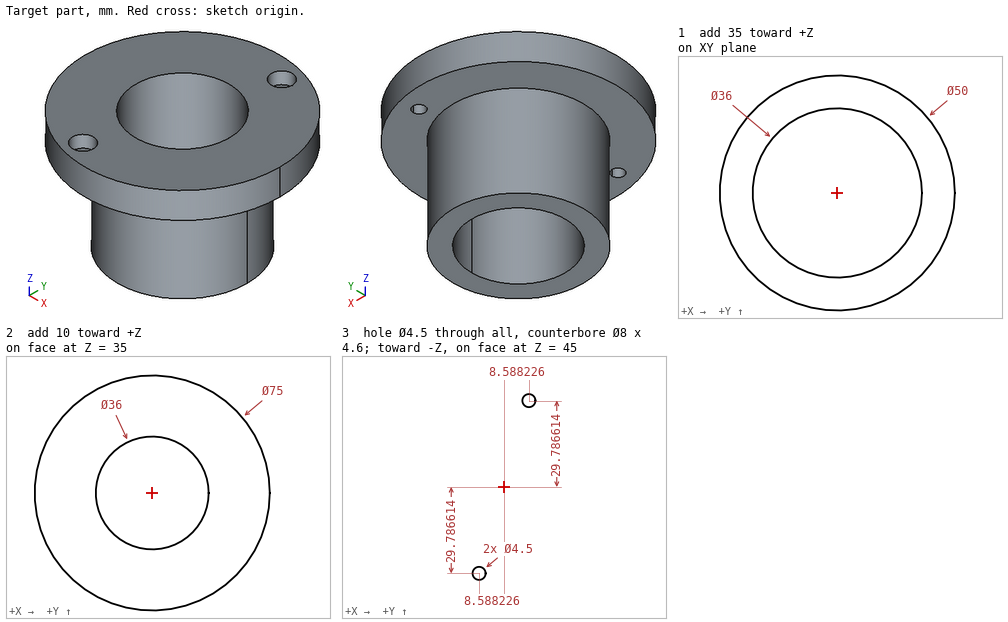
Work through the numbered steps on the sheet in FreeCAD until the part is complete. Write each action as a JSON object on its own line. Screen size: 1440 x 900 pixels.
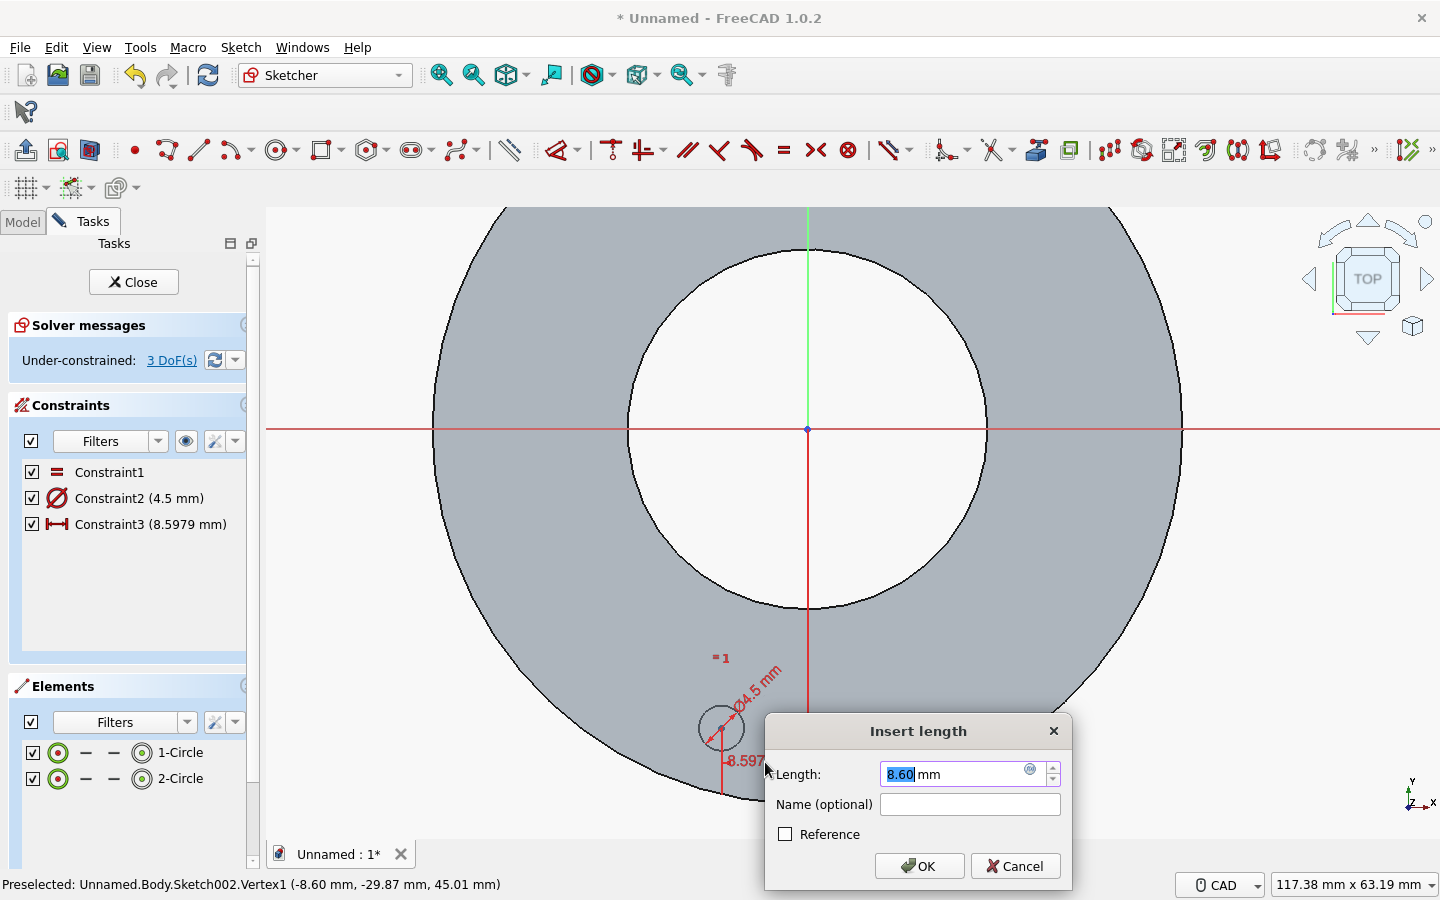
{"action": "type", "text": "8.588226"}
{"action": "key", "text": "Return"}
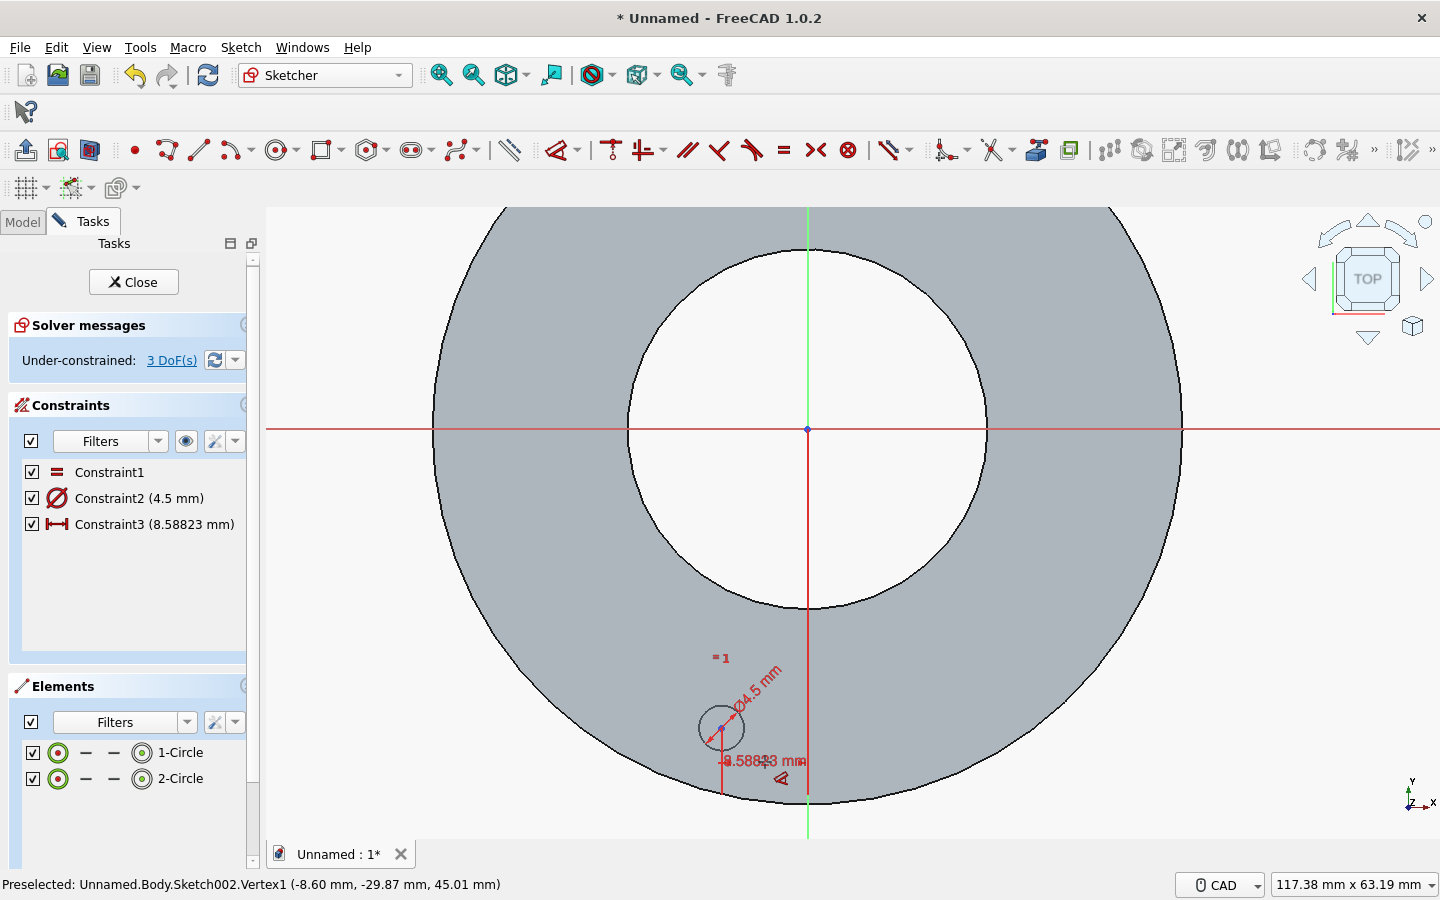
{"action": "scroll", "coordinate": [738, 713], "scroll_direction": "down", "scroll_amount": 2}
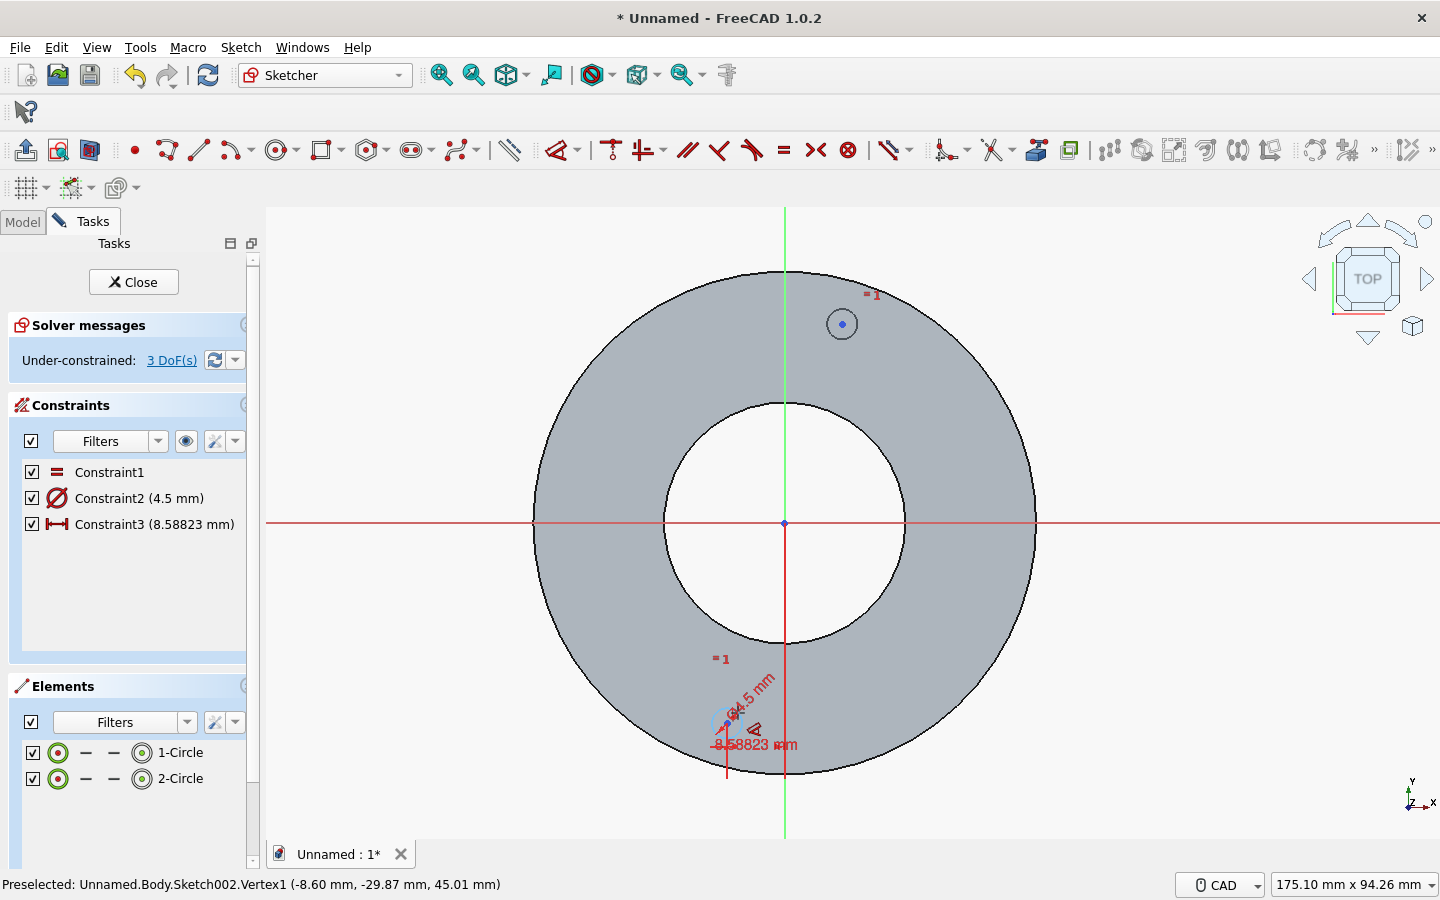
{"action": "left_click", "coordinate": [842, 324]}
{"action": "left_click", "coordinate": [813, 290]}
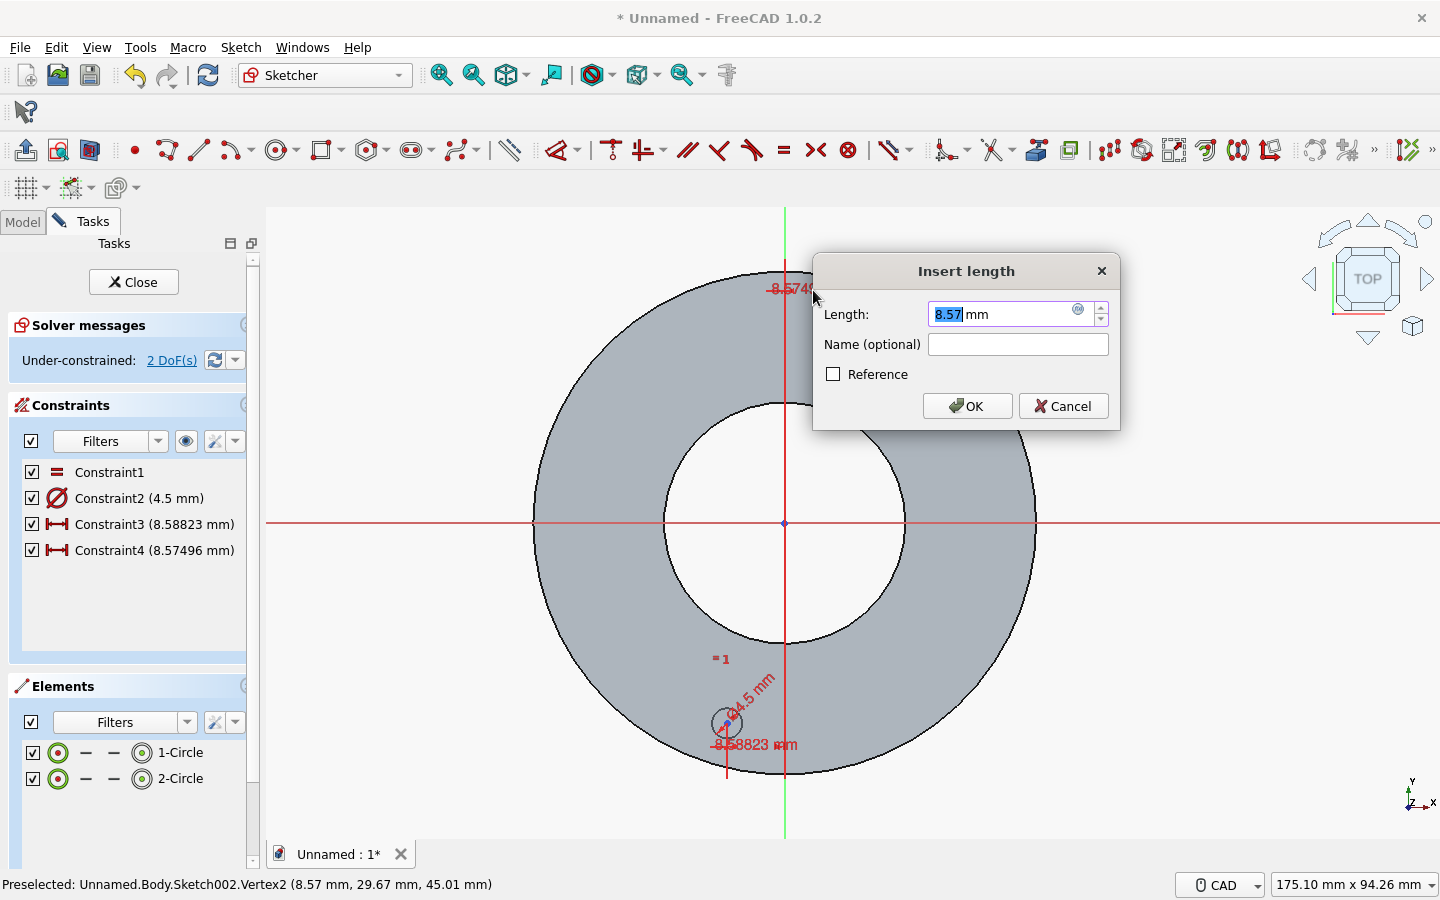
{"action": "type", "text": "8.588226"}
{"action": "key", "text": "Return"}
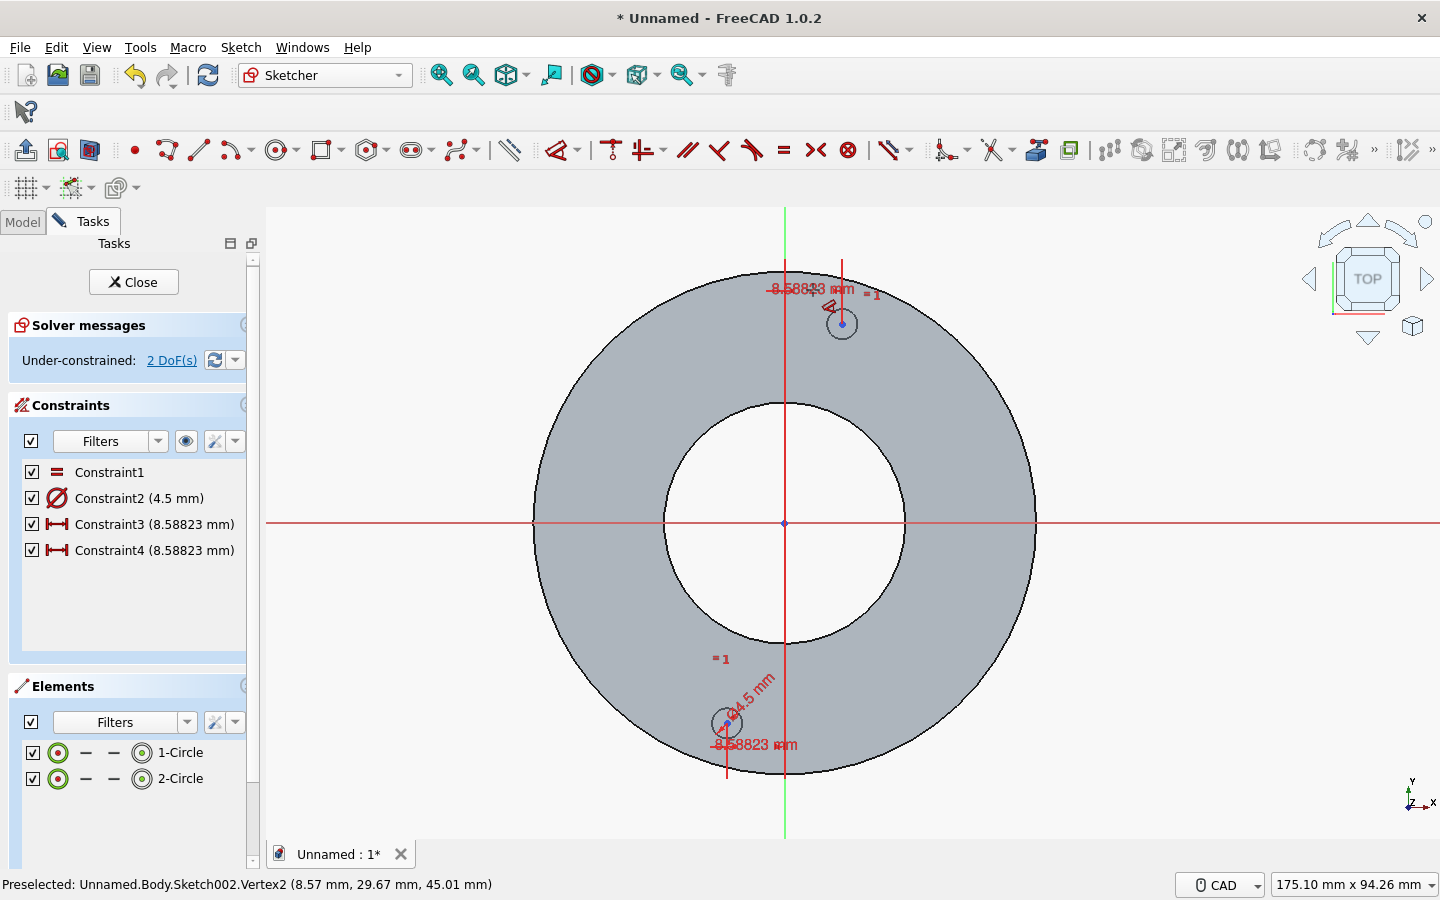
{"action": "left_click", "coordinate": [727, 723]}
{"action": "left_click", "coordinate": [693, 623]}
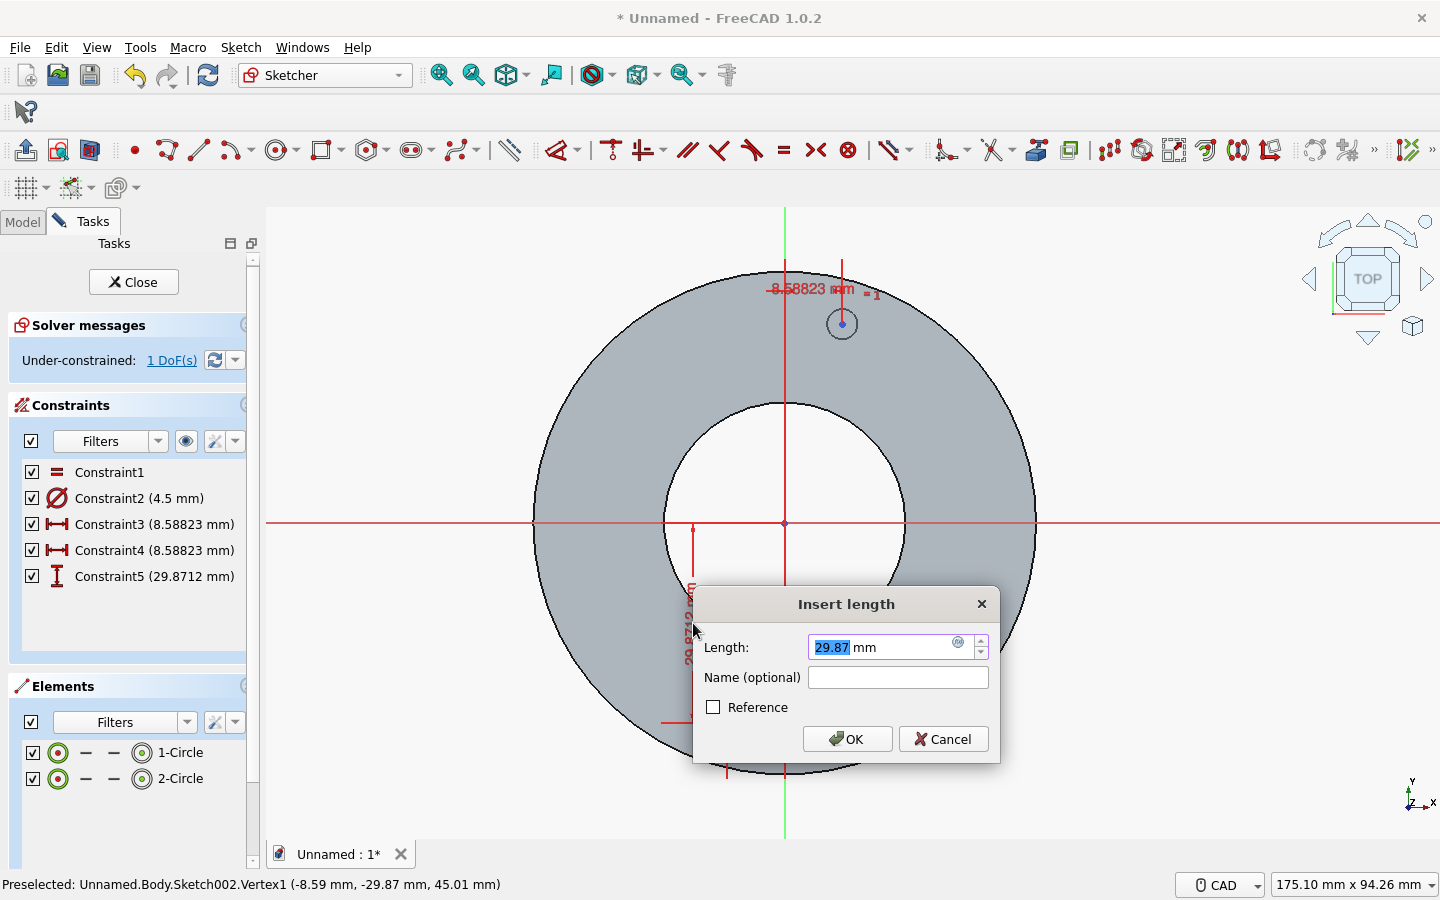
{"action": "type", "text": "29.786614"}
{"action": "key", "text": "Return"}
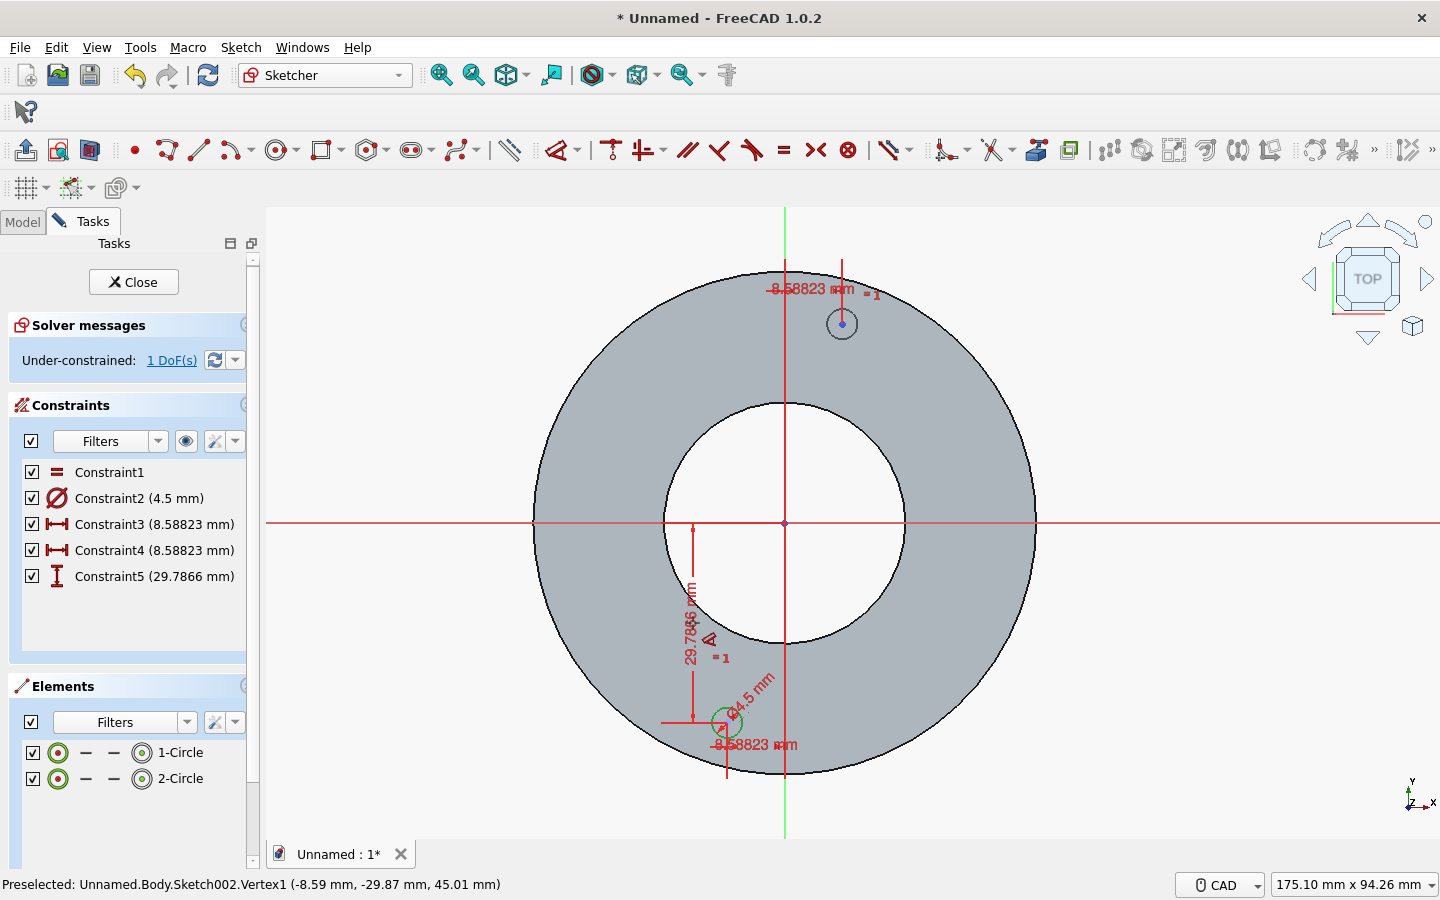
{"action": "left_click", "coordinate": [842, 324]}
{"action": "left_click", "coordinate": [876, 424]}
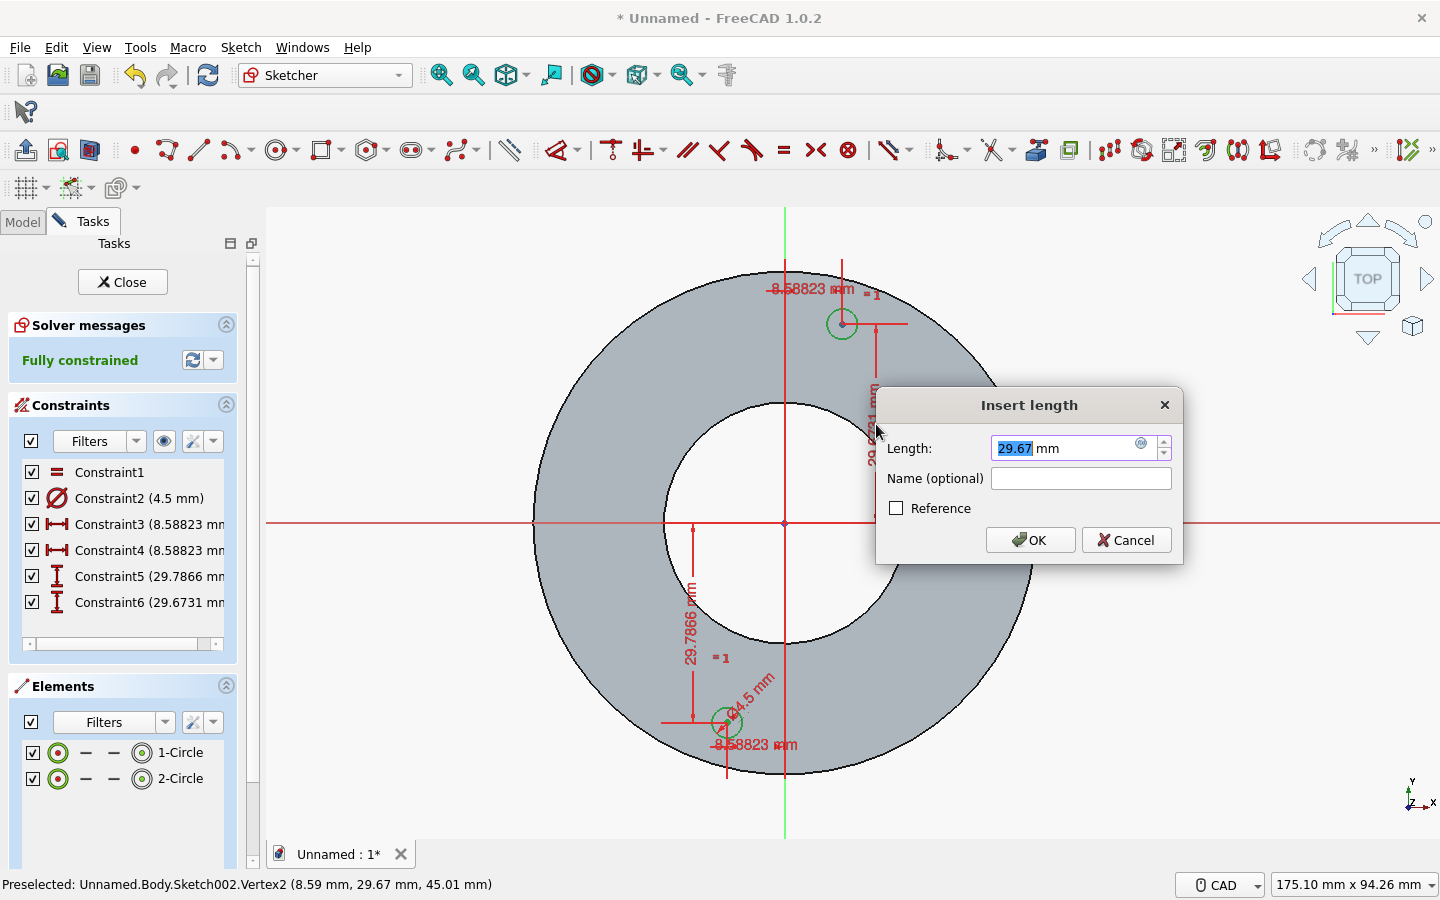
{"action": "type", "text": "29.786614"}
{"action": "key", "text": "Return"}
{"action": "key", "text": "Escape"}